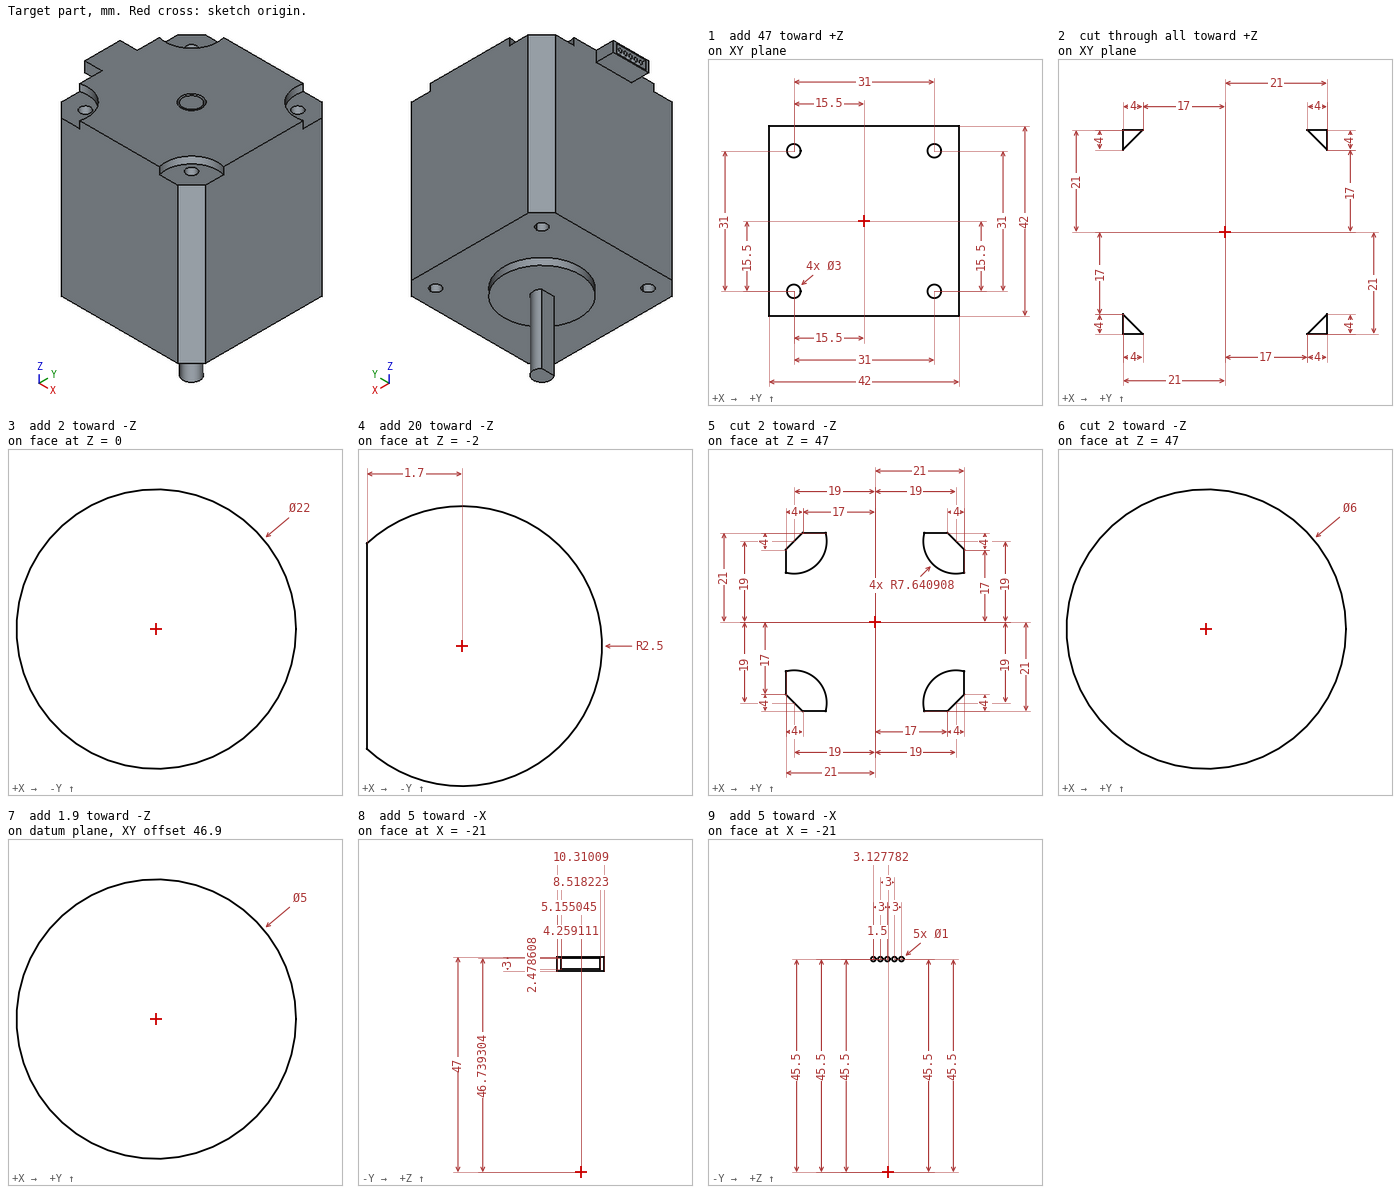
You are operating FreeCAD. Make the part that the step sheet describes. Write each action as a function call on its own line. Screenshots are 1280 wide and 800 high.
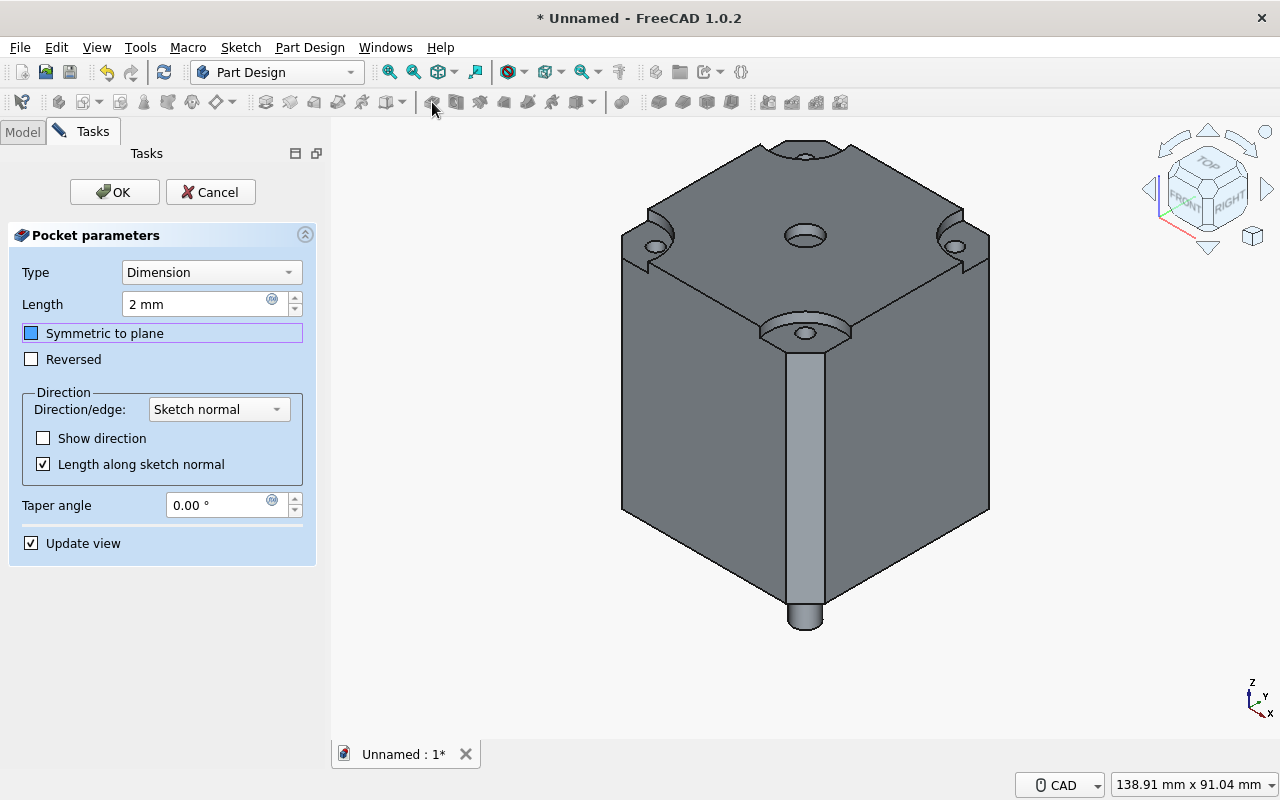
click(115, 192)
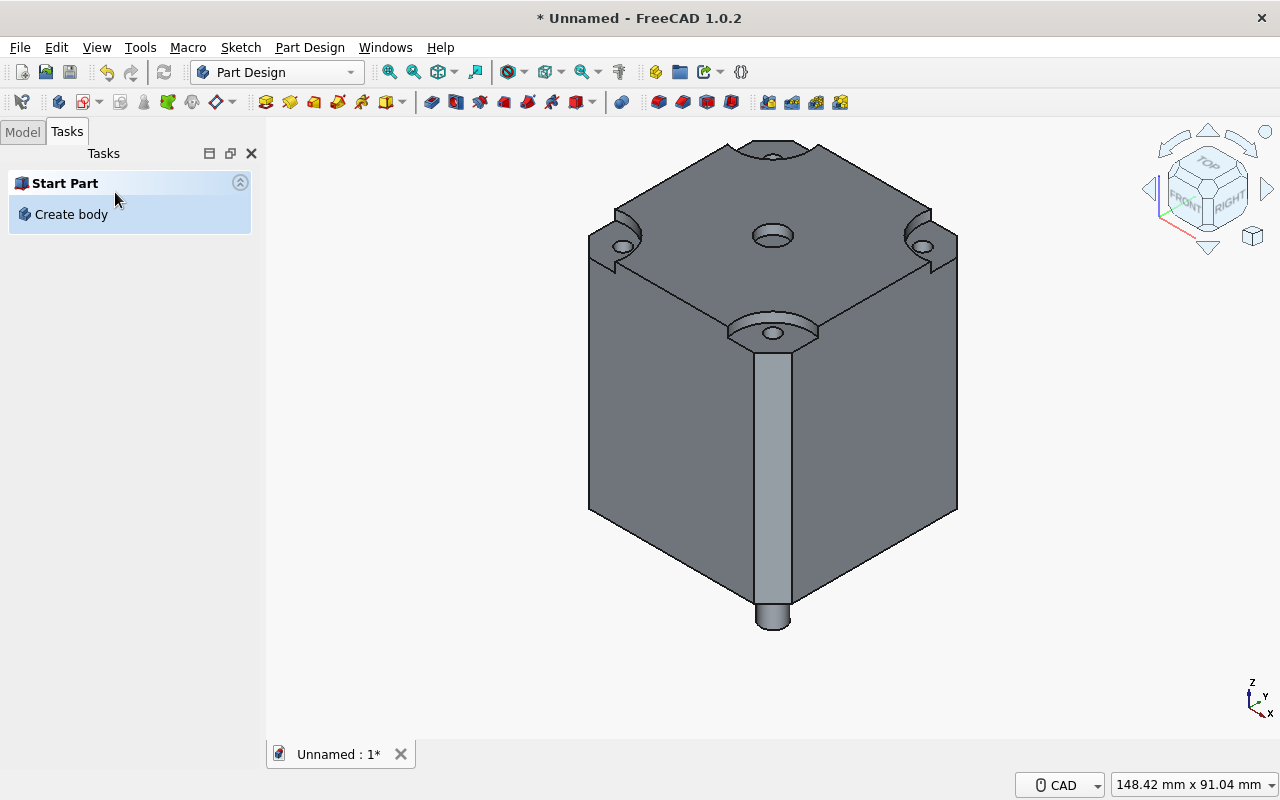
click(23, 131)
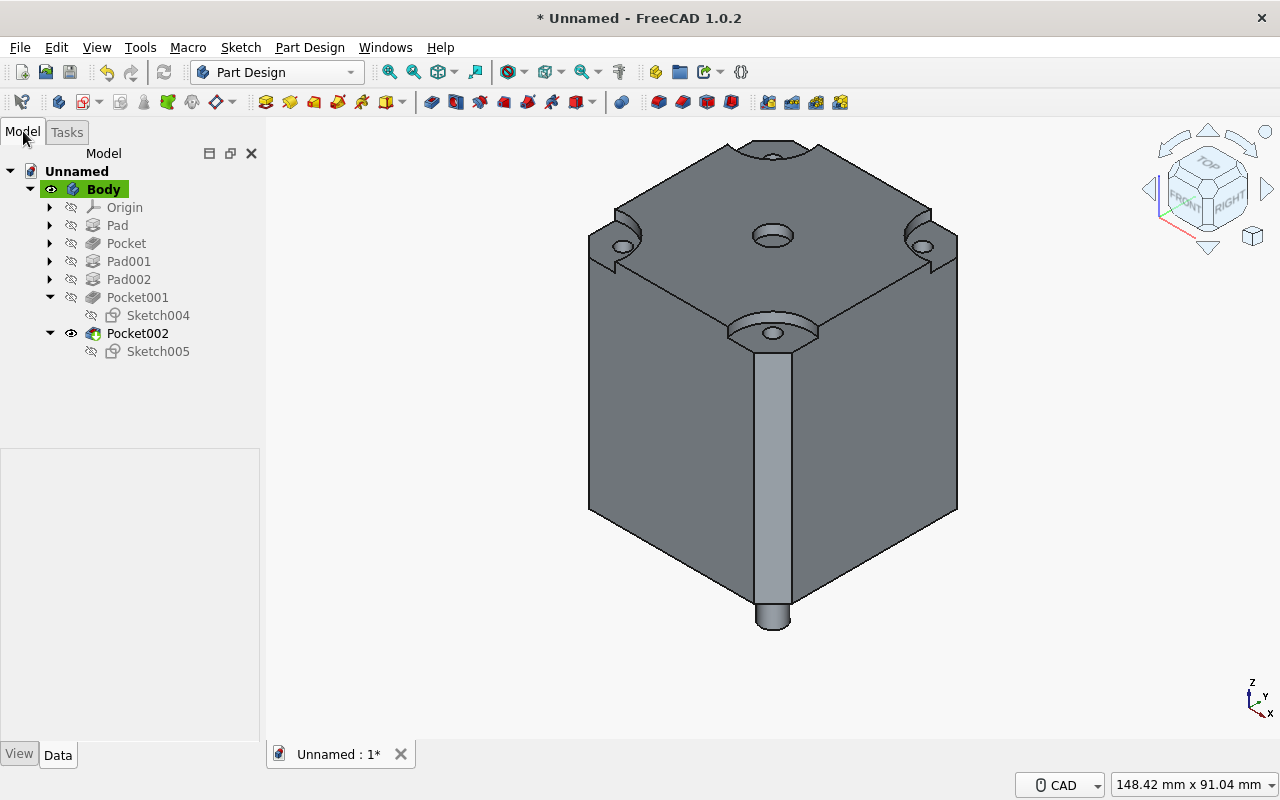
click(50, 207)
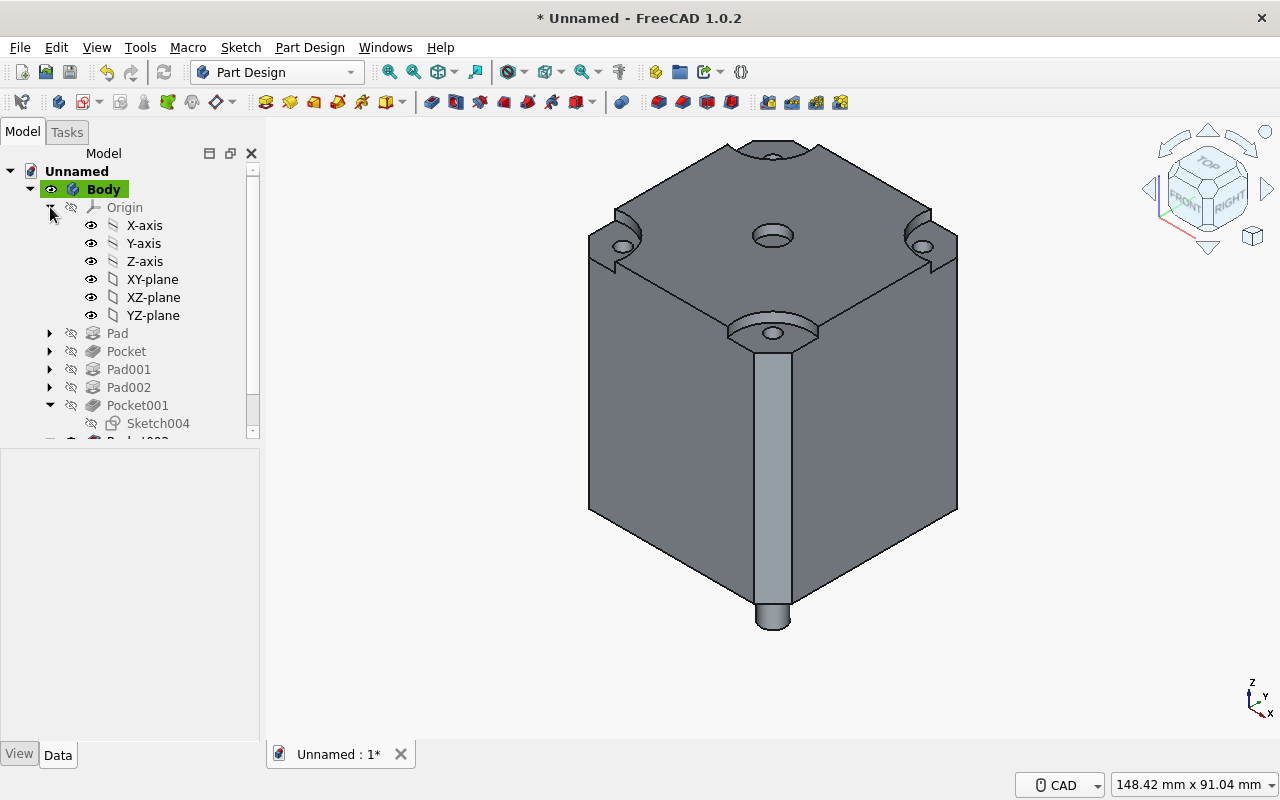
click(136, 279)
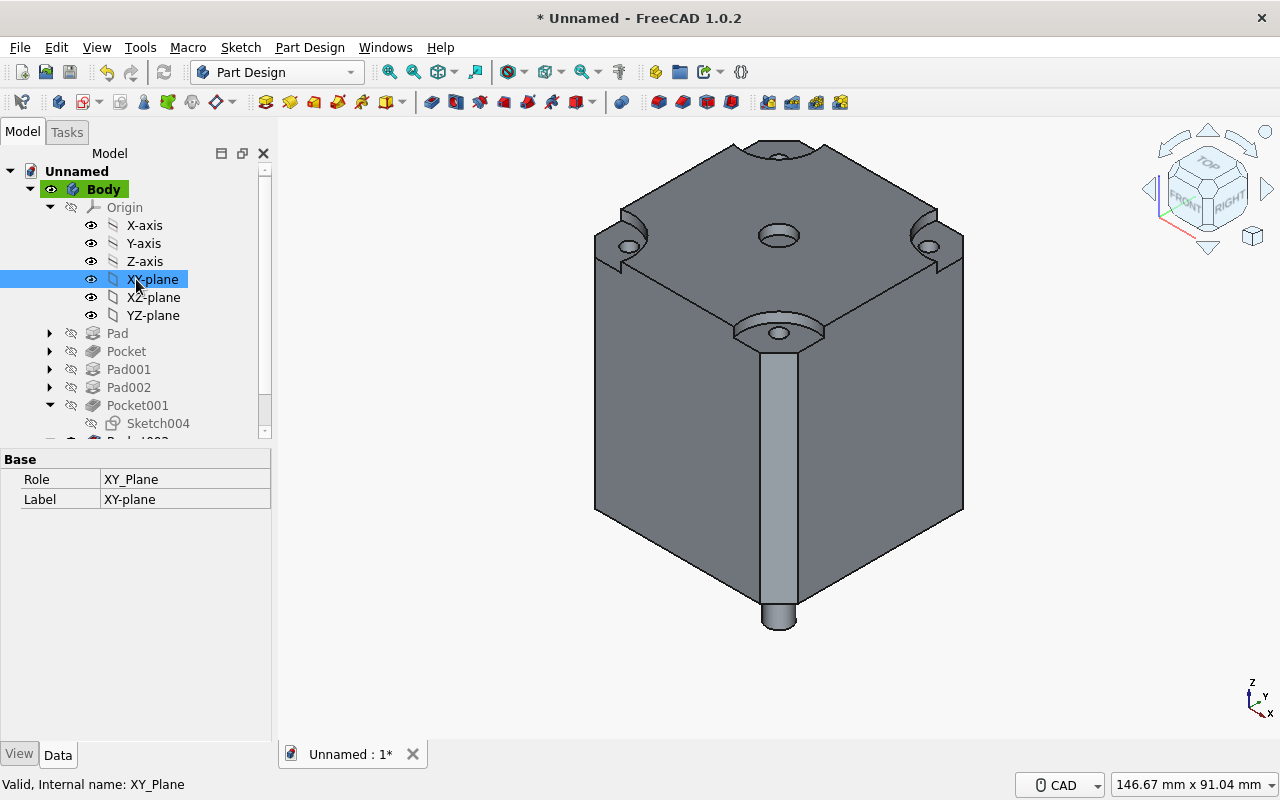
click(216, 102)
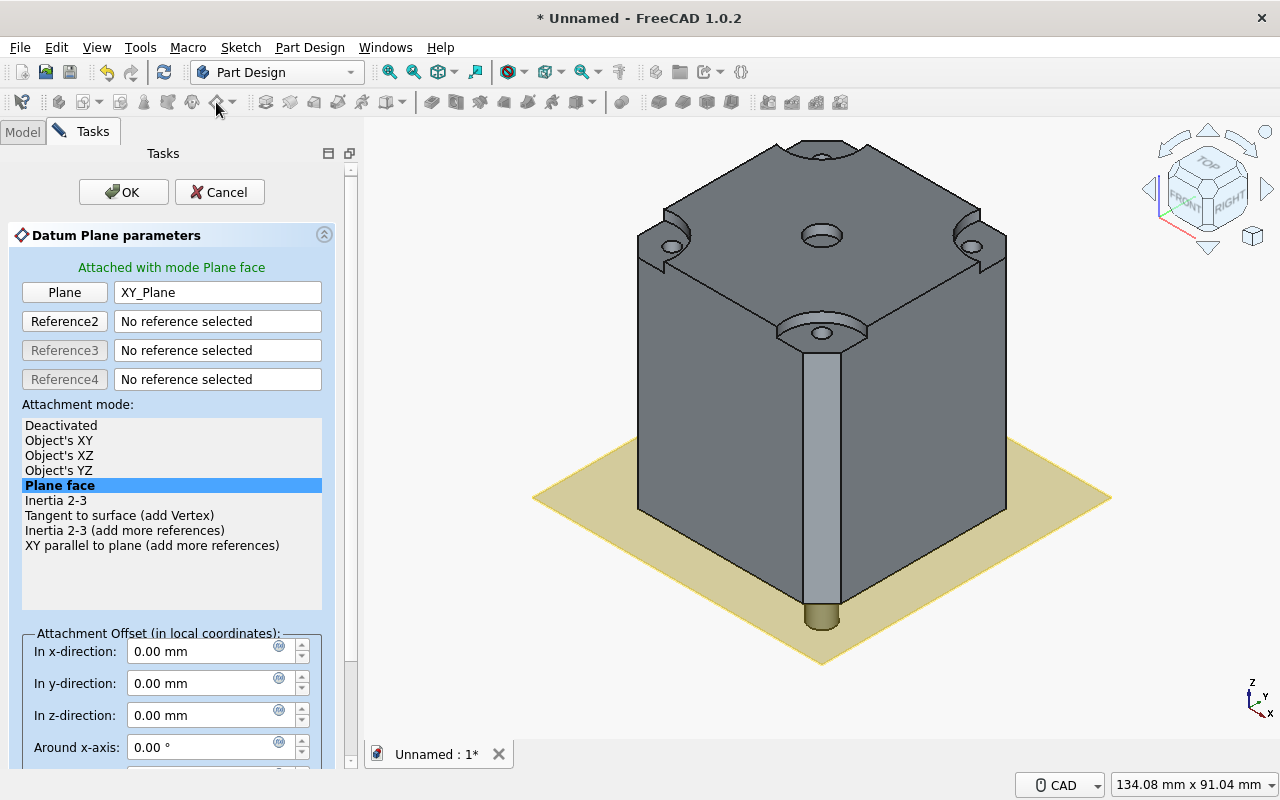
triple_click(210, 715)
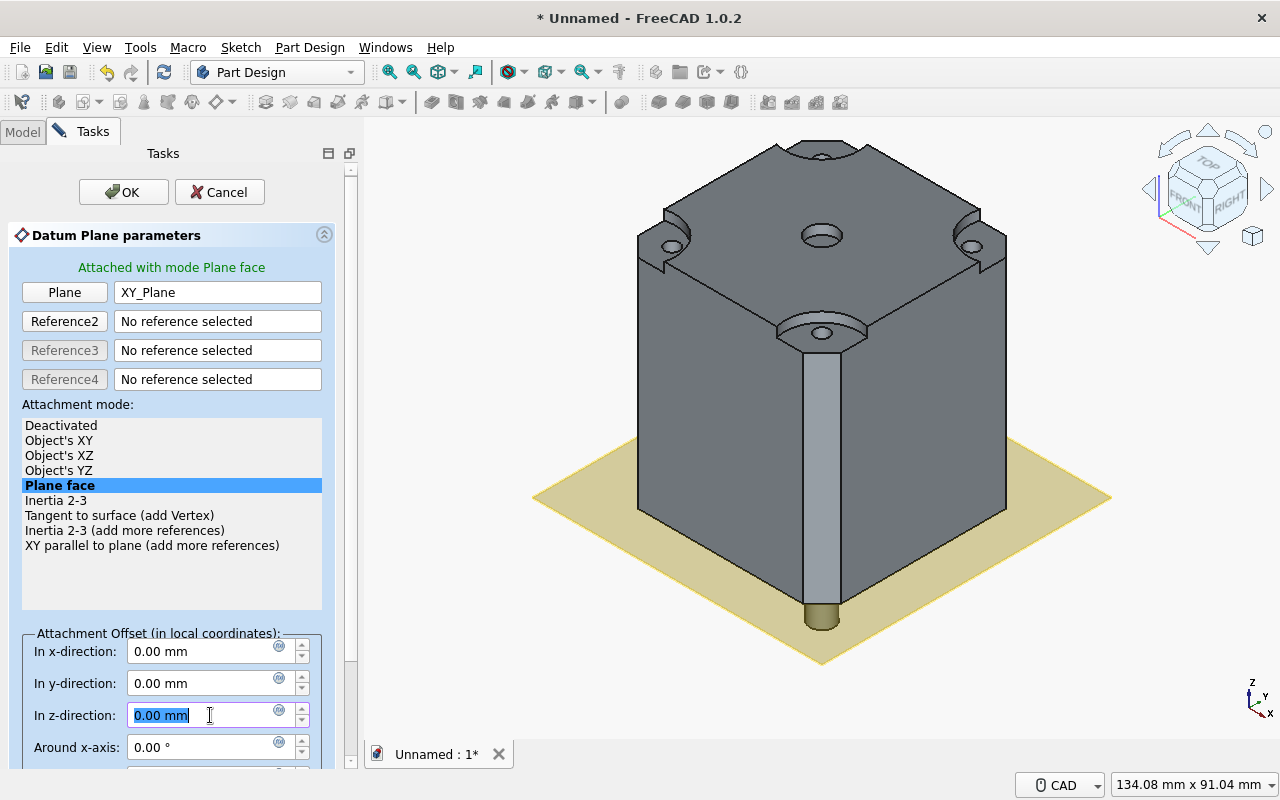
text(46.9)
key(Tab)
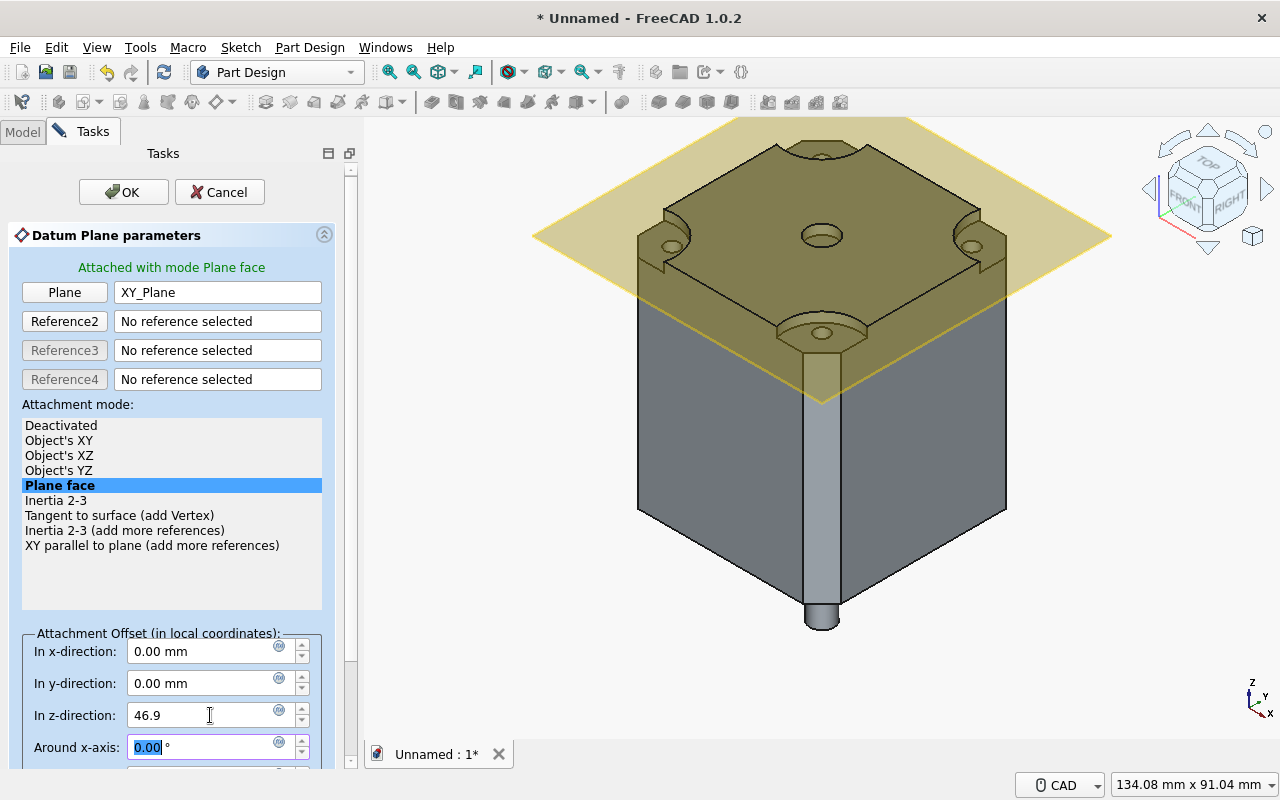
click(124, 192)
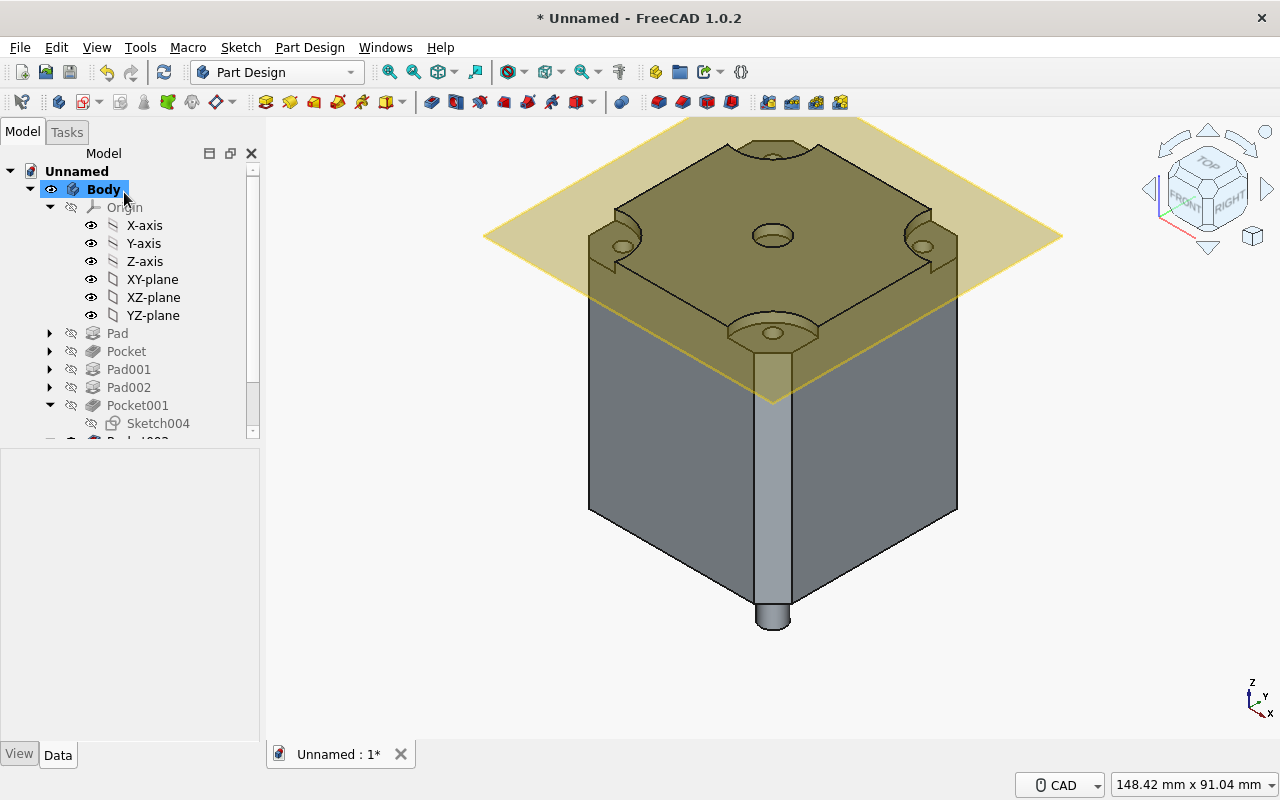
scroll(100, 293, down, 3)